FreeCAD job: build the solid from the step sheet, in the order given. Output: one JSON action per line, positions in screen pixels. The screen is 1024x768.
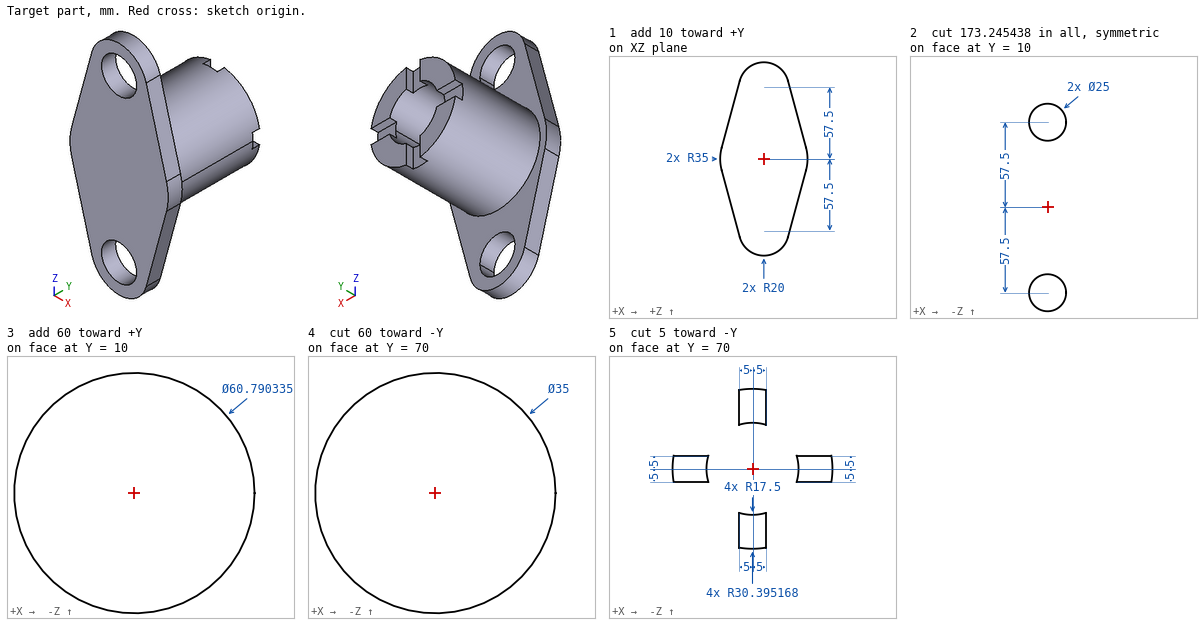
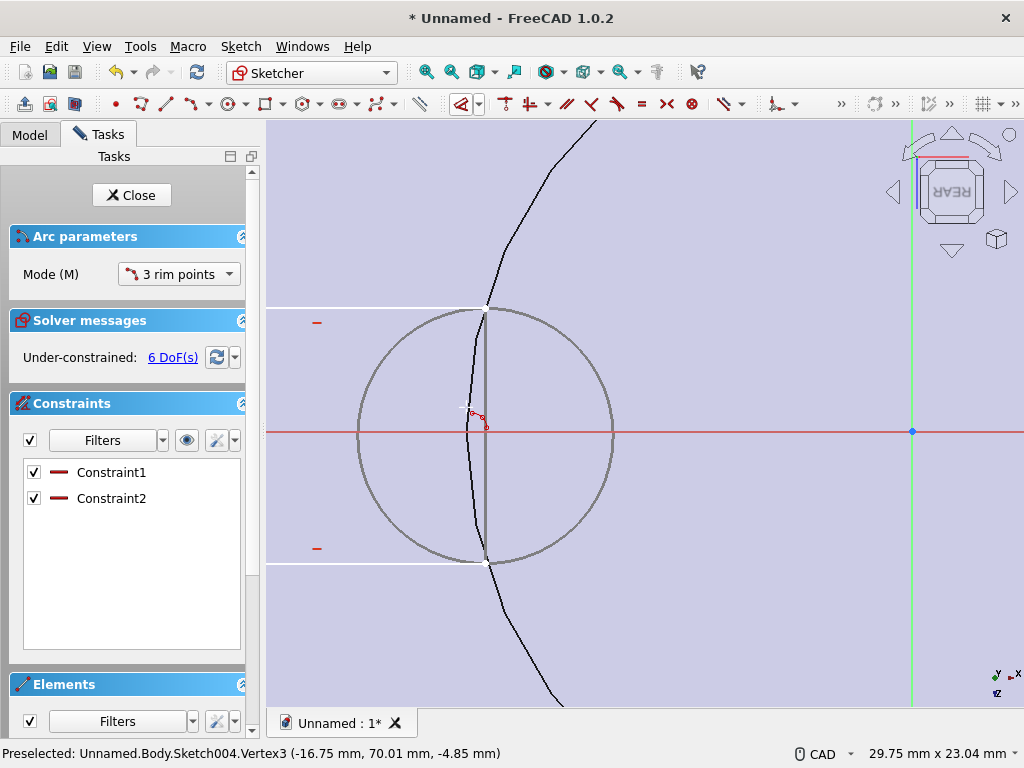
{"action": "left_click", "coordinate": [467, 406]}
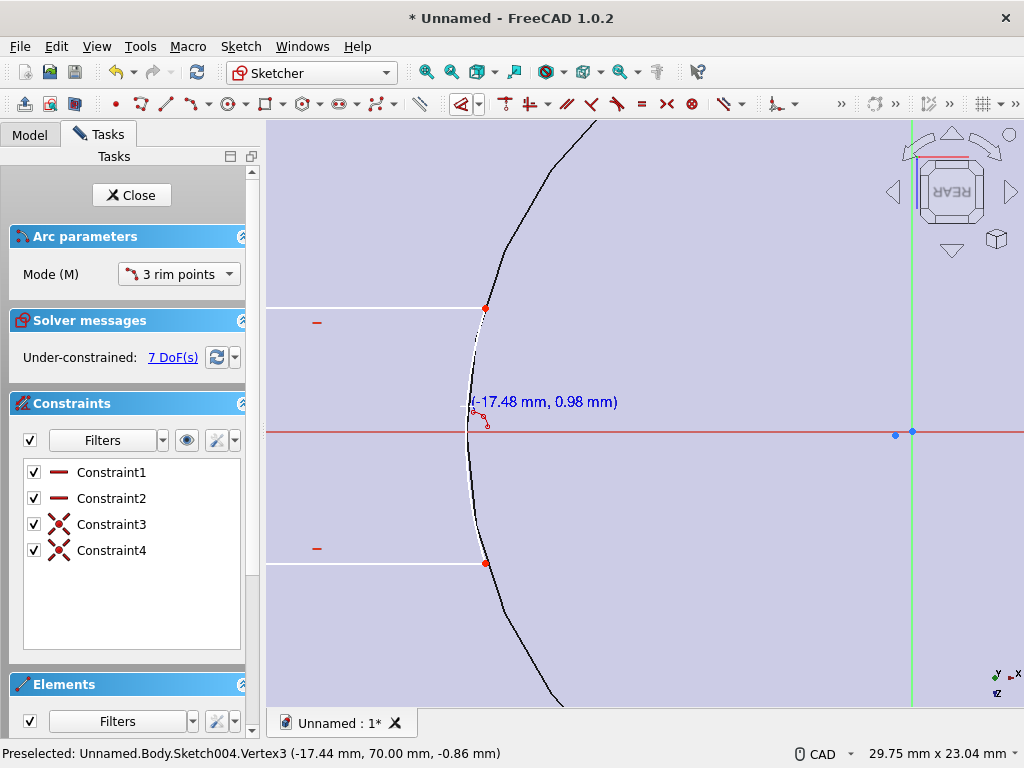
{"action": "scroll", "coordinate": [467, 407], "scroll_direction": "down", "scroll_amount": 7}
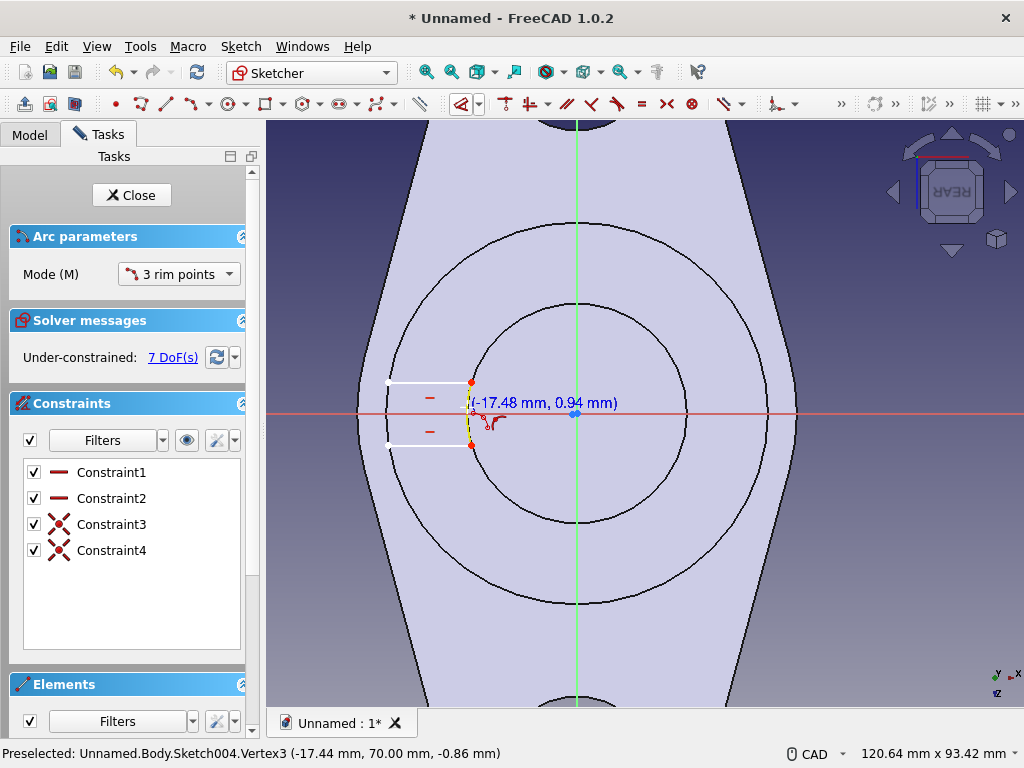
{"action": "left_click", "coordinate": [389, 383]}
{"action": "left_click", "coordinate": [389, 446]}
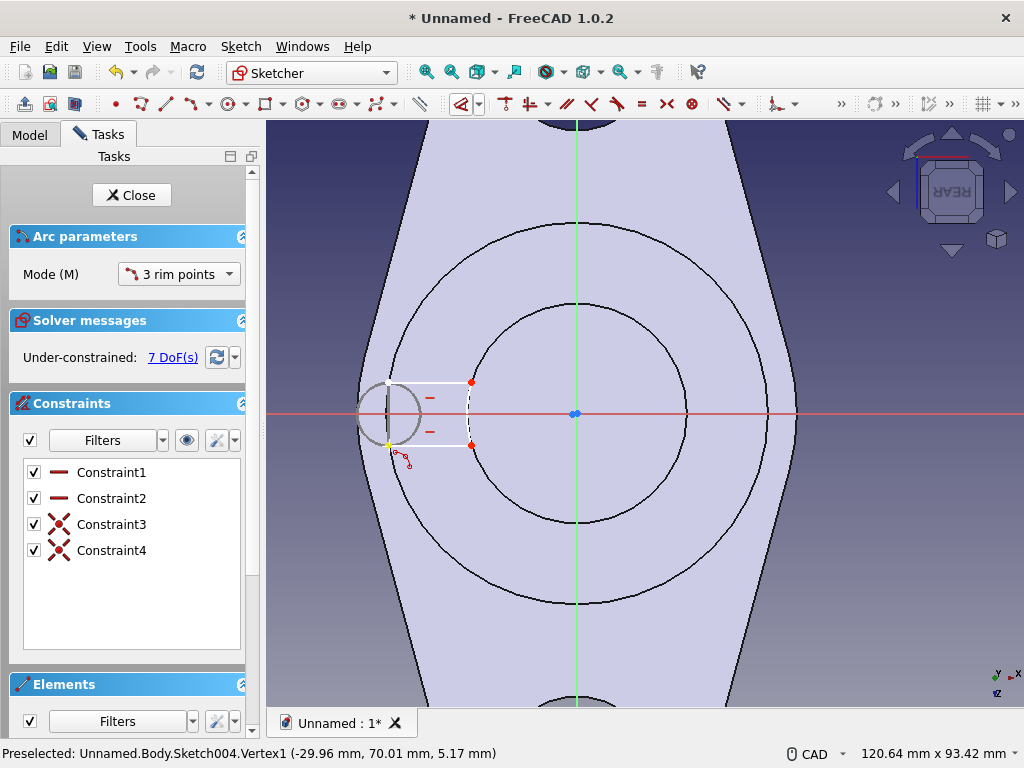
{"action": "scroll", "coordinate": [386, 407], "scroll_direction": "up", "scroll_amount": 10}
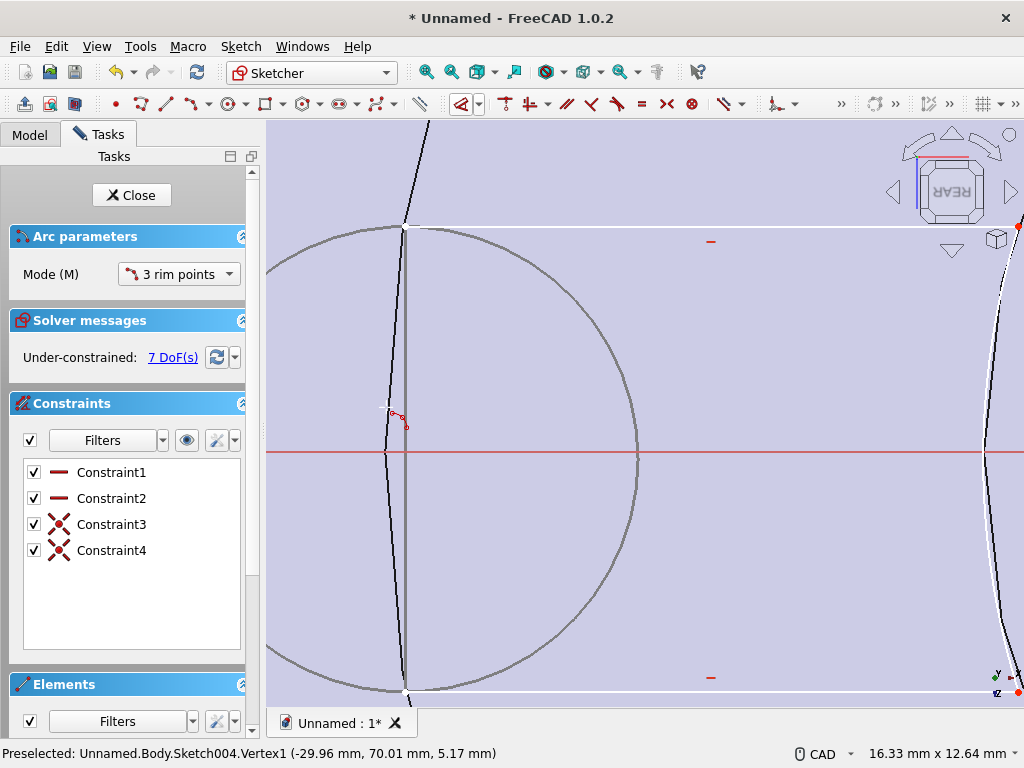
{"action": "left_click", "coordinate": [386, 405]}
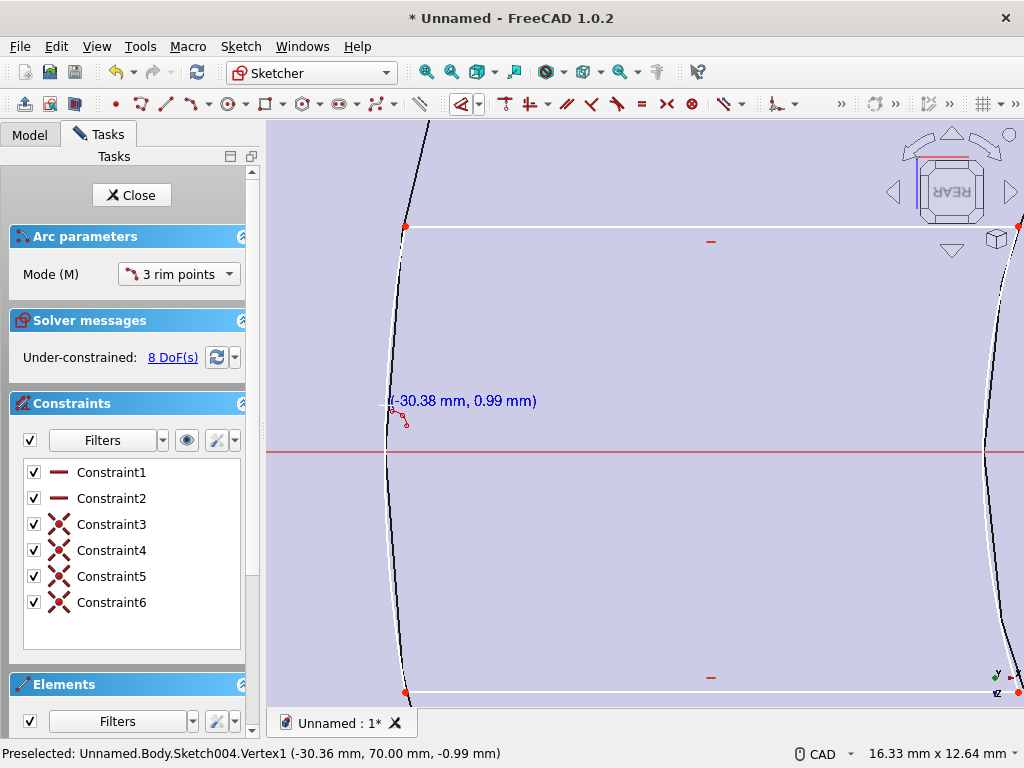
{"action": "left_click", "coordinate": [166, 104]}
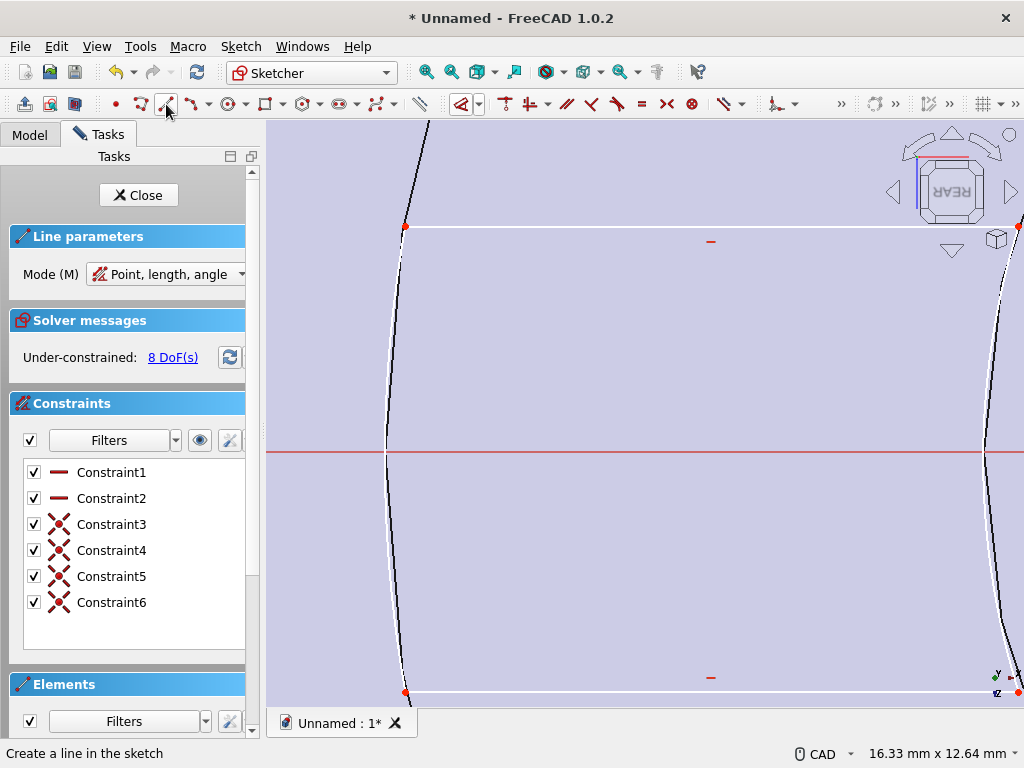
{"action": "scroll", "coordinate": [386, 407], "scroll_direction": "down", "scroll_amount": 10}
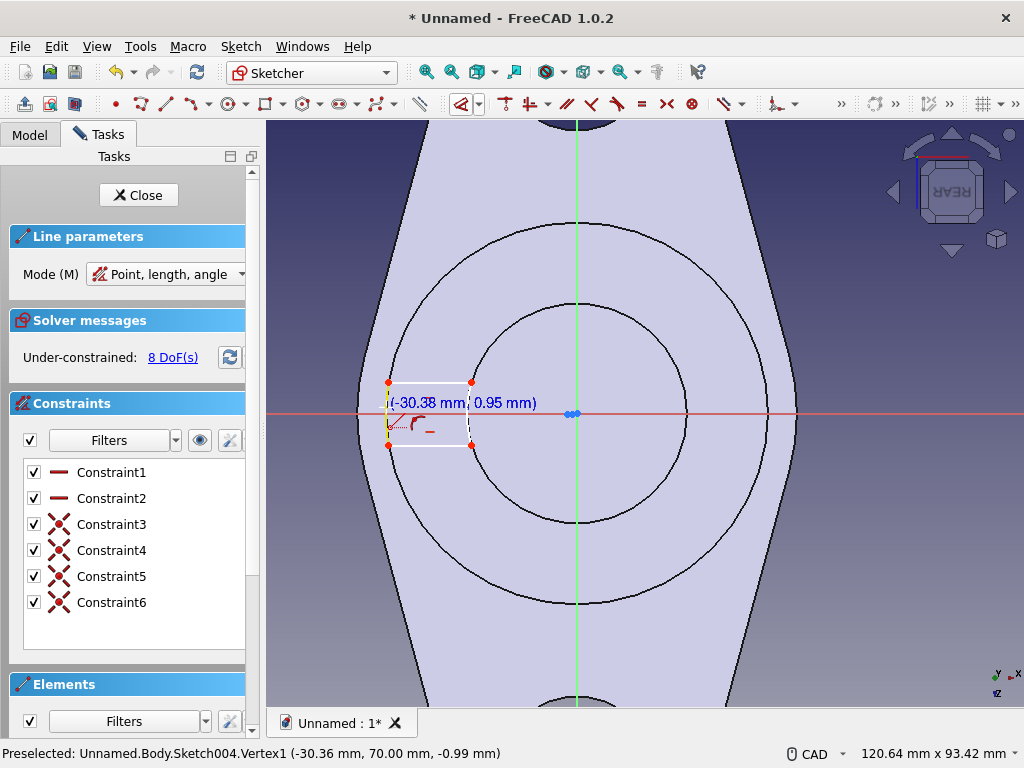
{"action": "left_click", "coordinate": [546, 519]}
{"action": "left_click", "coordinate": [546, 602]}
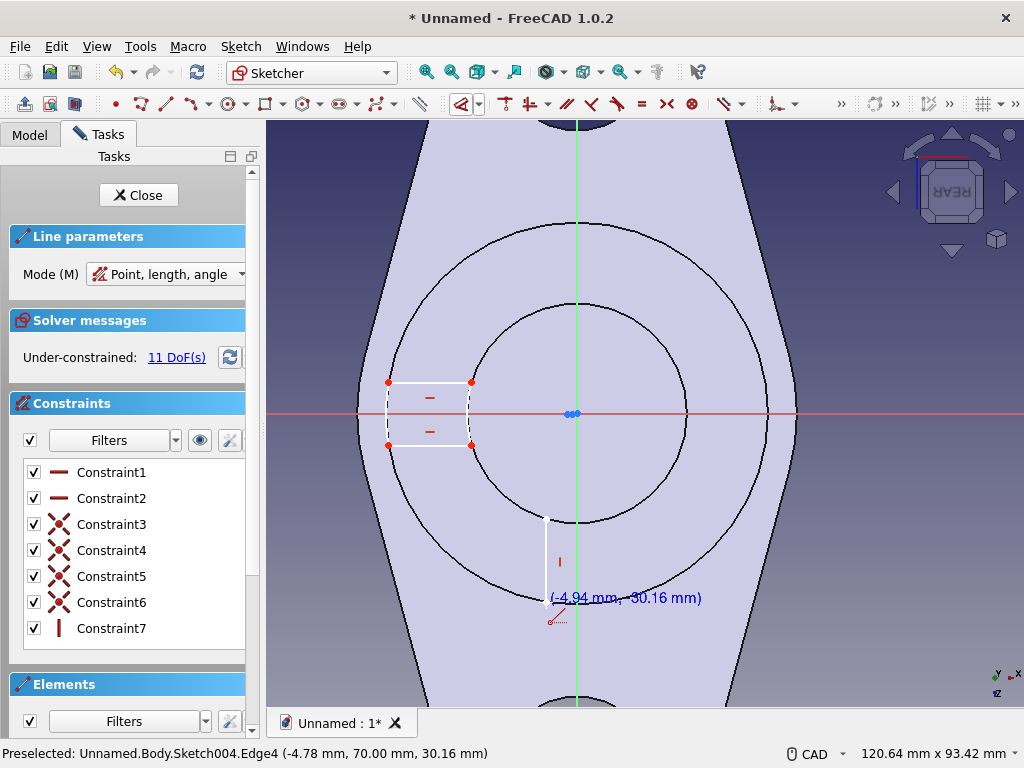
{"action": "left_click", "coordinate": [608, 602]}
{"action": "left_click", "coordinate": [608, 519]}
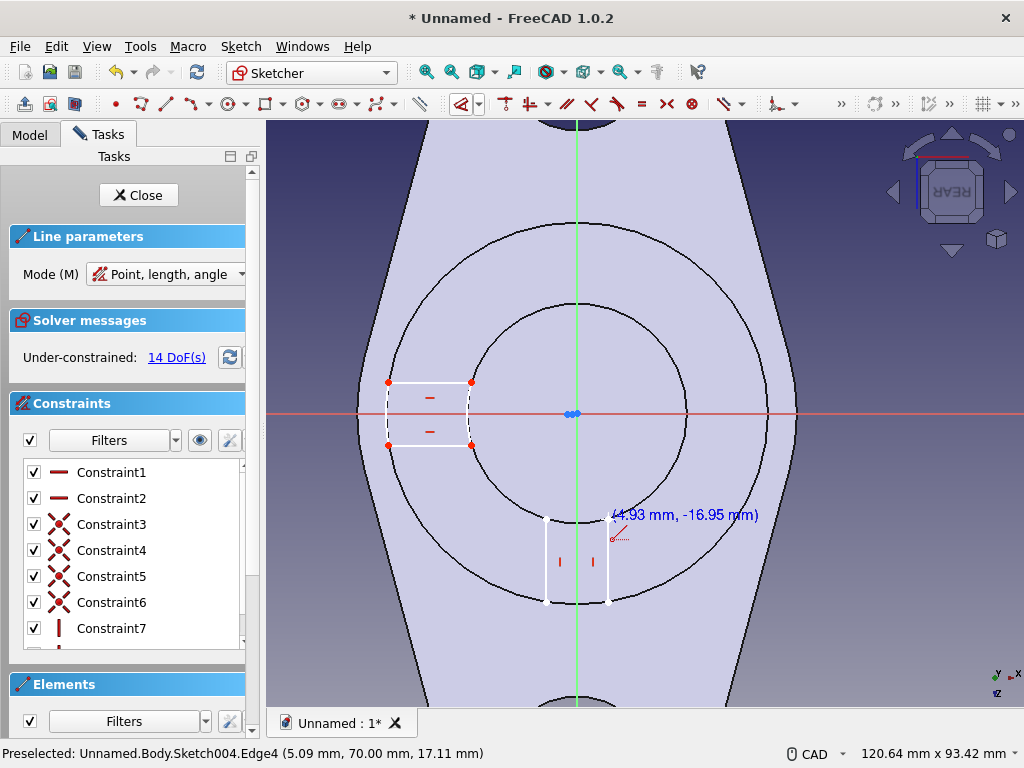
{"action": "left_click", "coordinate": [190, 104]}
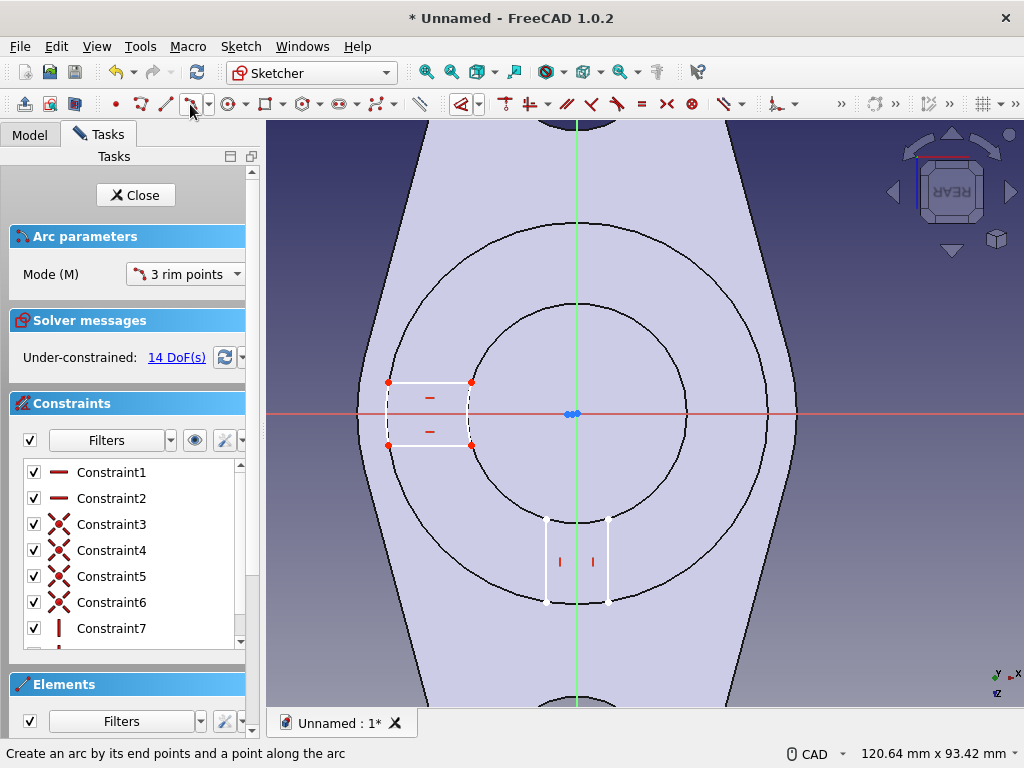
{"action": "left_click", "coordinate": [546, 603]}
{"action": "left_click", "coordinate": [608, 603]}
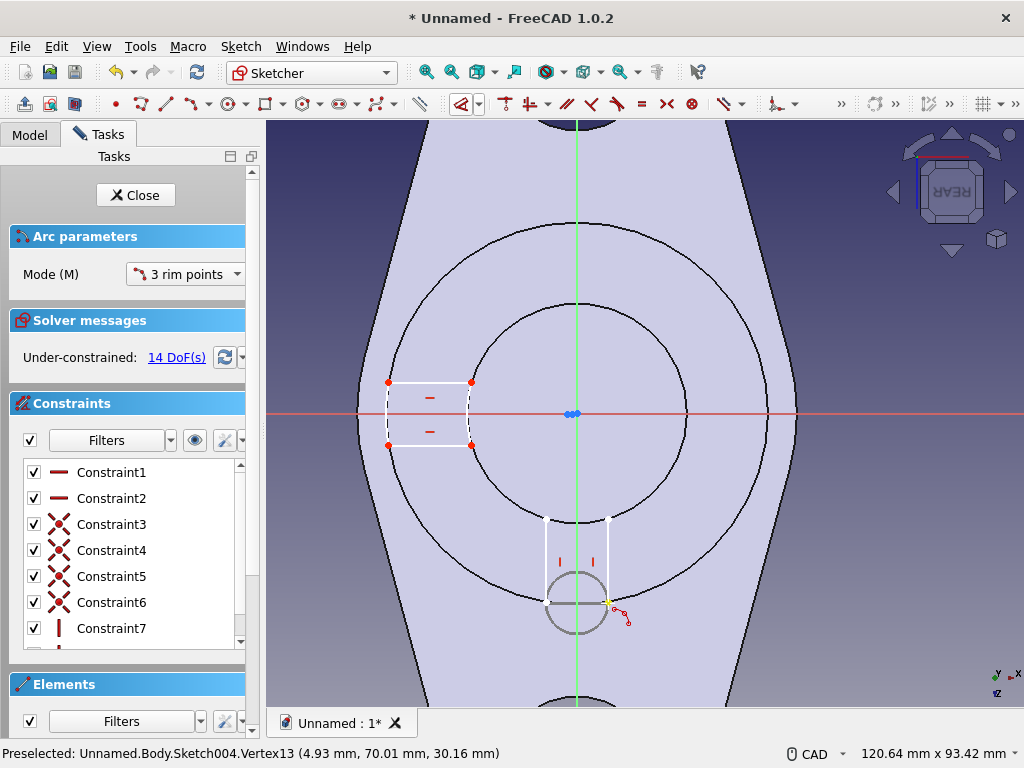
{"action": "scroll", "coordinate": [571, 604], "scroll_direction": "up", "scroll_amount": 10}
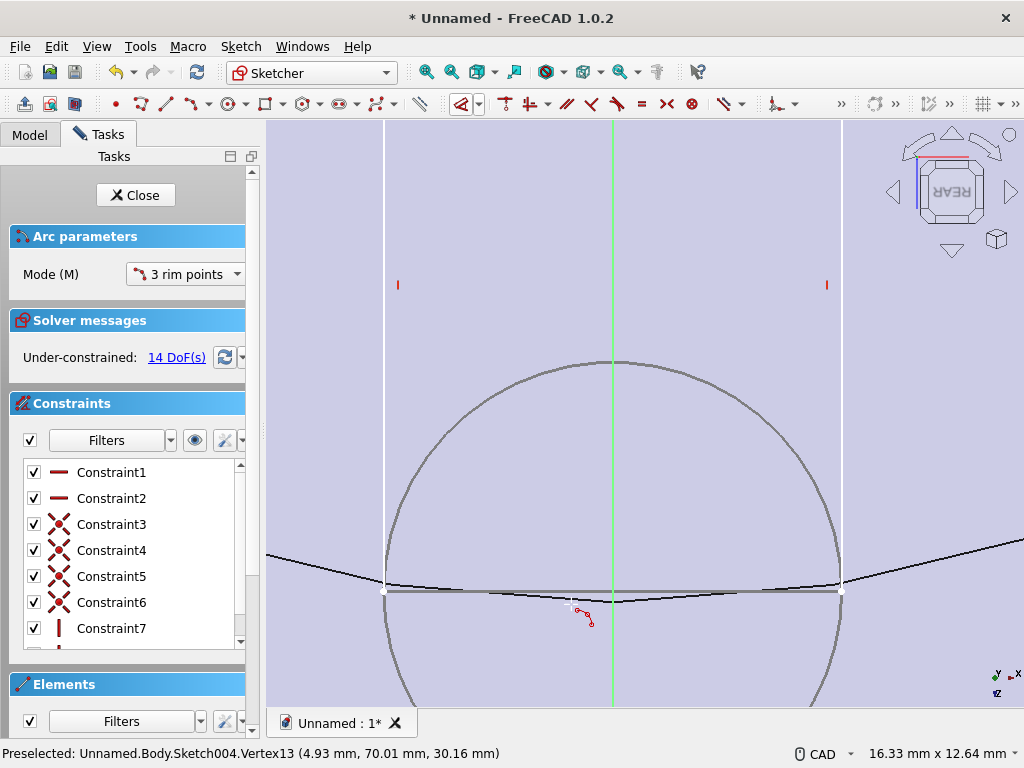
{"action": "left_click", "coordinate": [566, 601]}